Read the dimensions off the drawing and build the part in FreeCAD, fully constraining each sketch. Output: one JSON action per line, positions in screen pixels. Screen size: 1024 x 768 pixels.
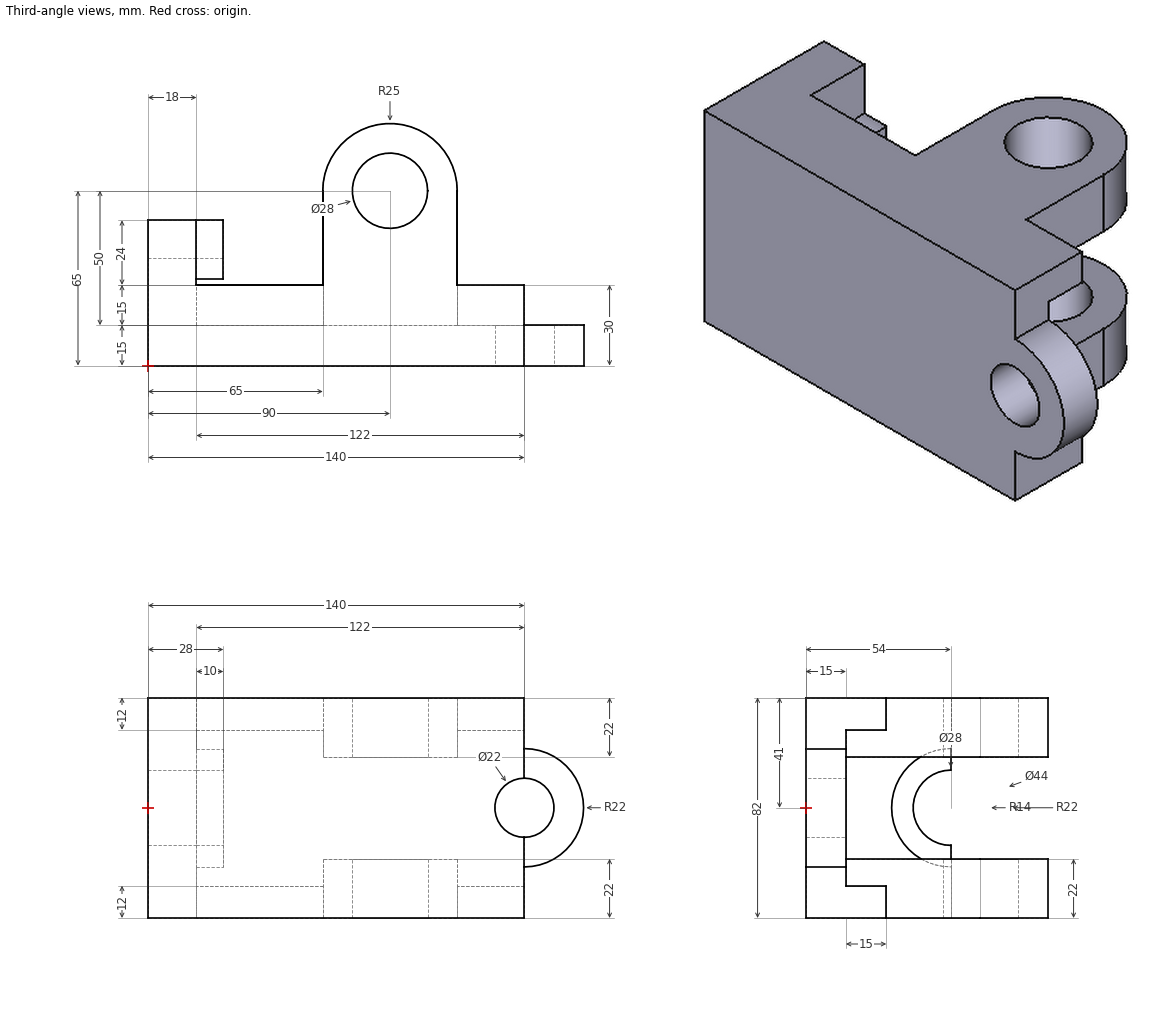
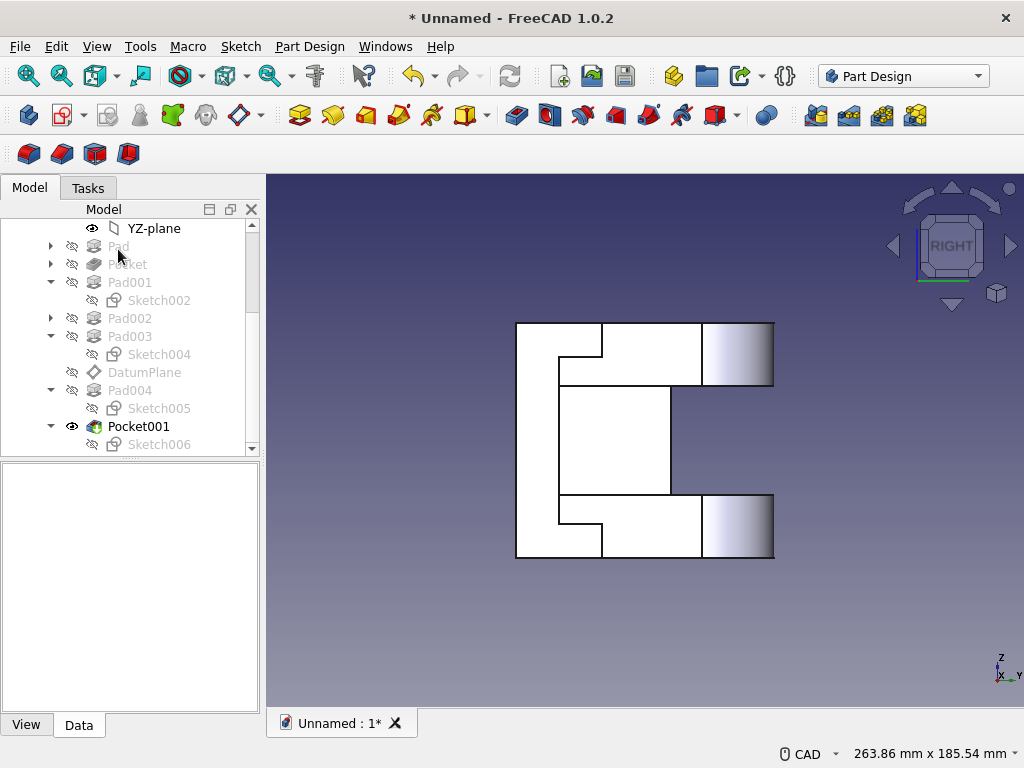
{"action": "left_click", "coordinate": [615, 439]}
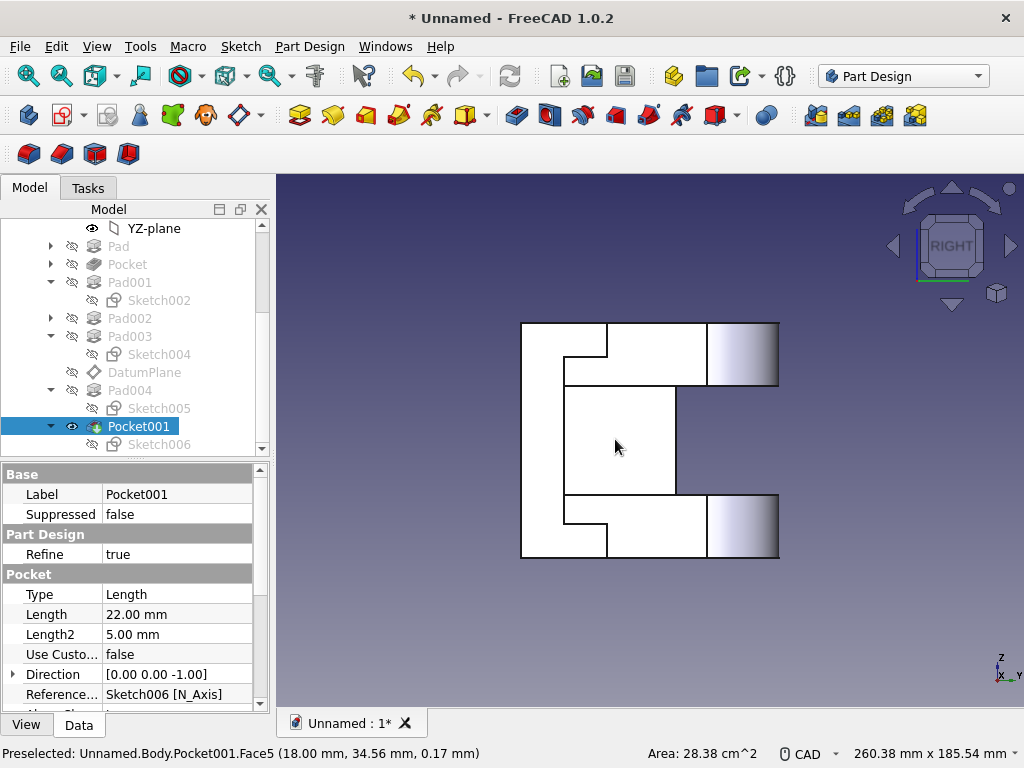
{"action": "left_click", "coordinate": [62, 116]}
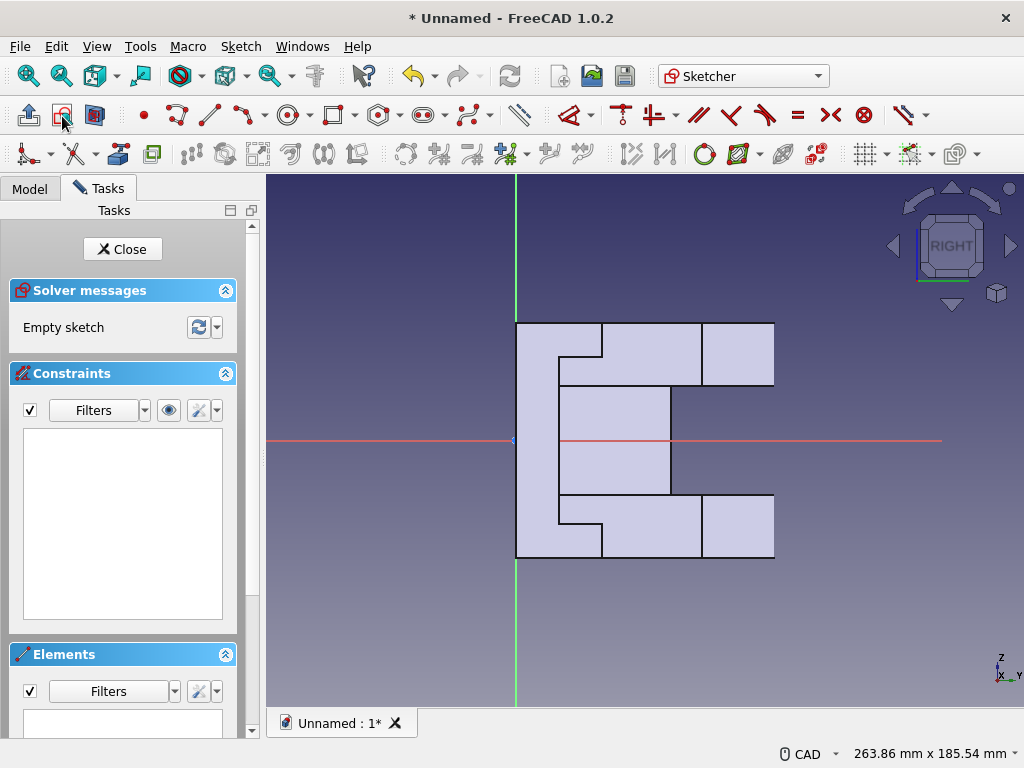
{"action": "scroll", "coordinate": [684, 441], "scroll_direction": "up", "scroll_amount": 3}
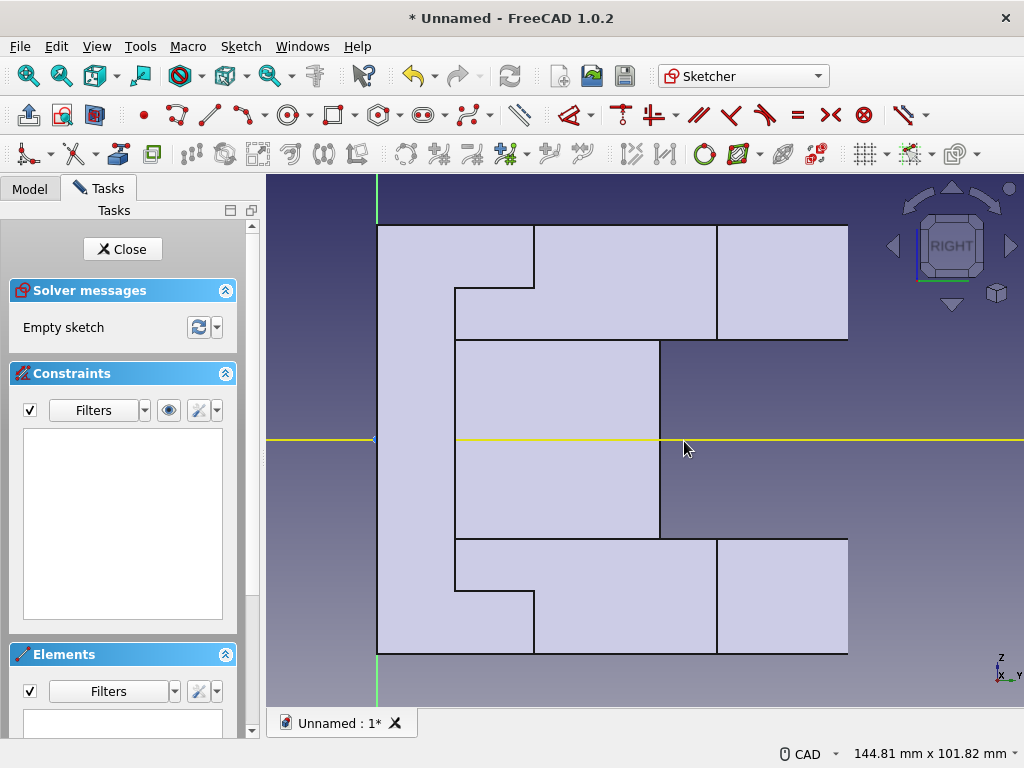
{"action": "left_click", "coordinate": [288, 116]}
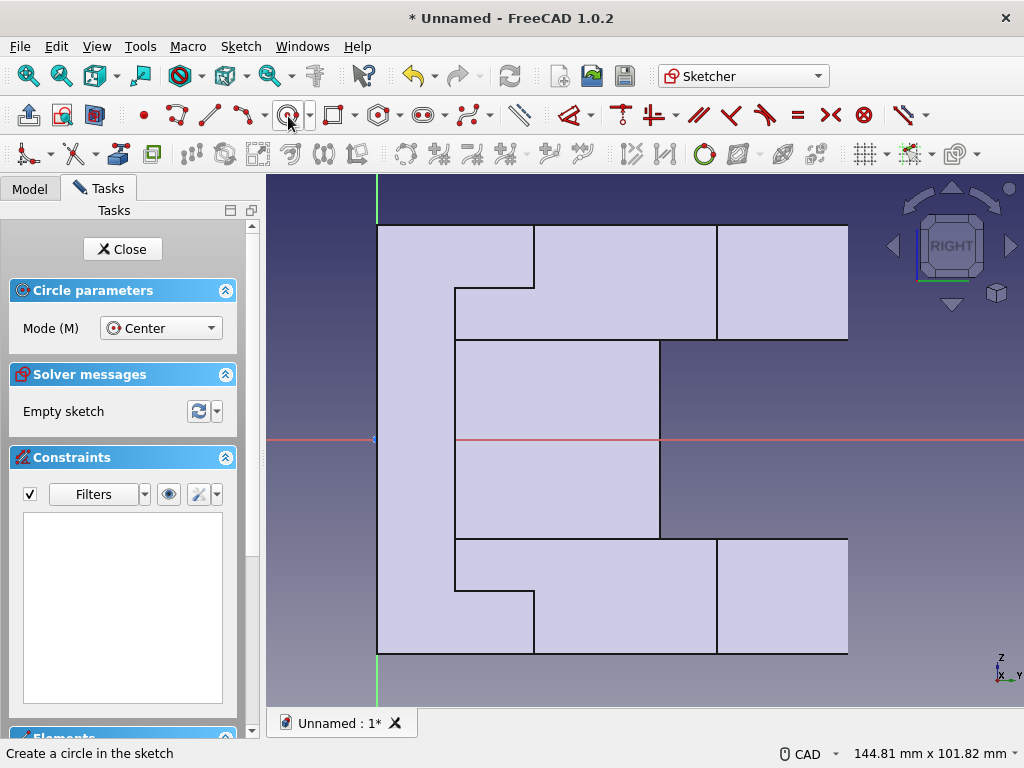
{"action": "left_click", "coordinate": [660, 440]}
{"action": "left_click", "coordinate": [741, 358]}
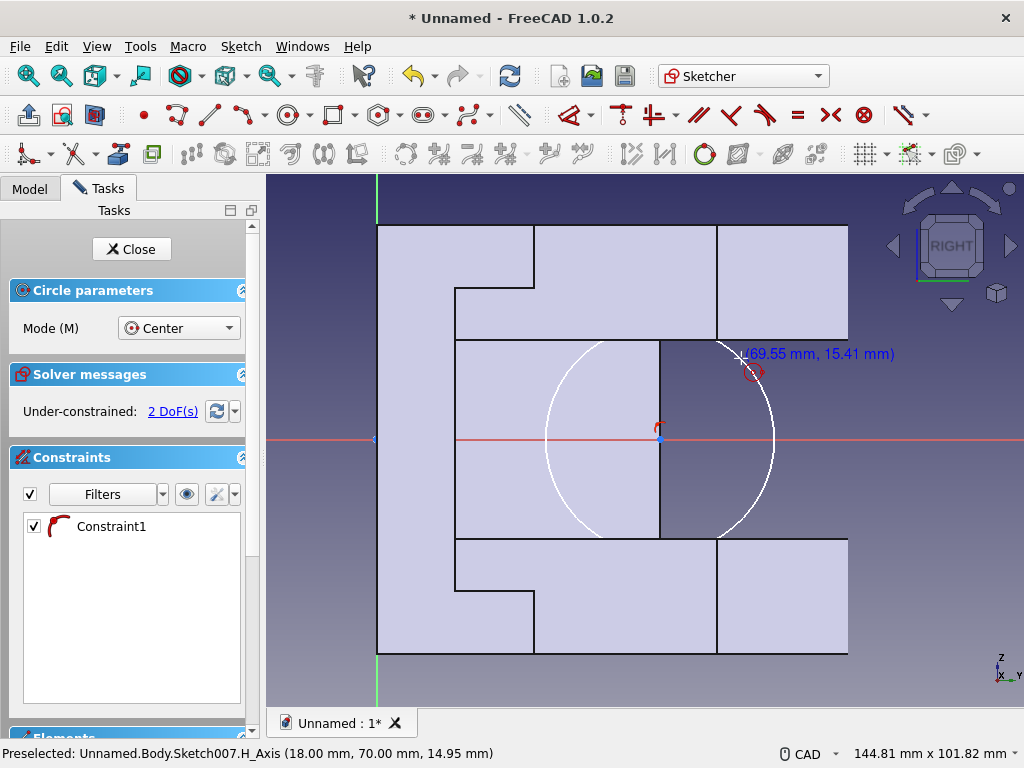
{"action": "left_click", "coordinate": [660, 440]}
{"action": "left_click", "coordinate": [711, 388]}
{"action": "key", "text": "Escape"}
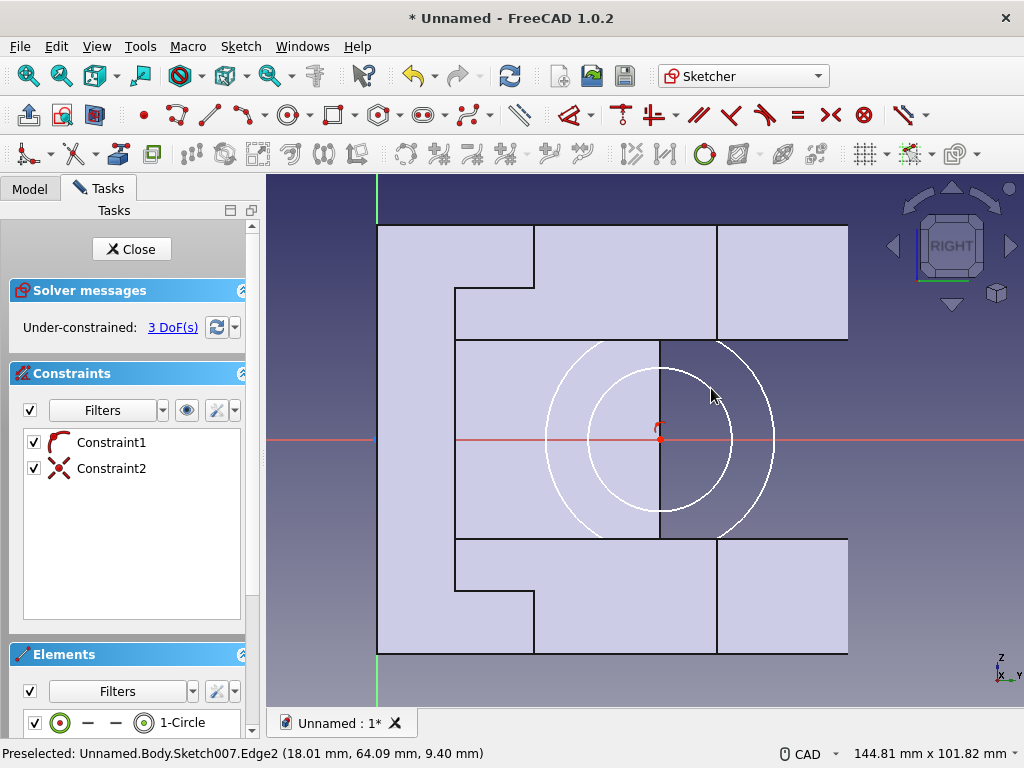
{"action": "key", "text": "d"}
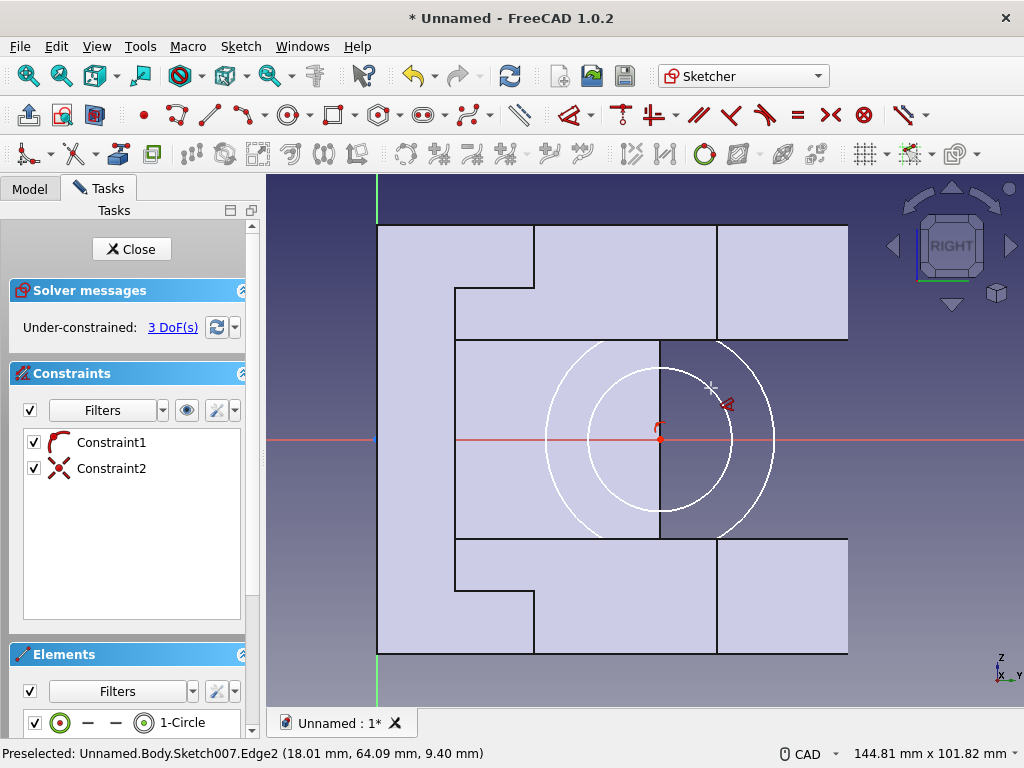
{"action": "left_click", "coordinate": [741, 359]}
{"action": "left_click", "coordinate": [764, 336]}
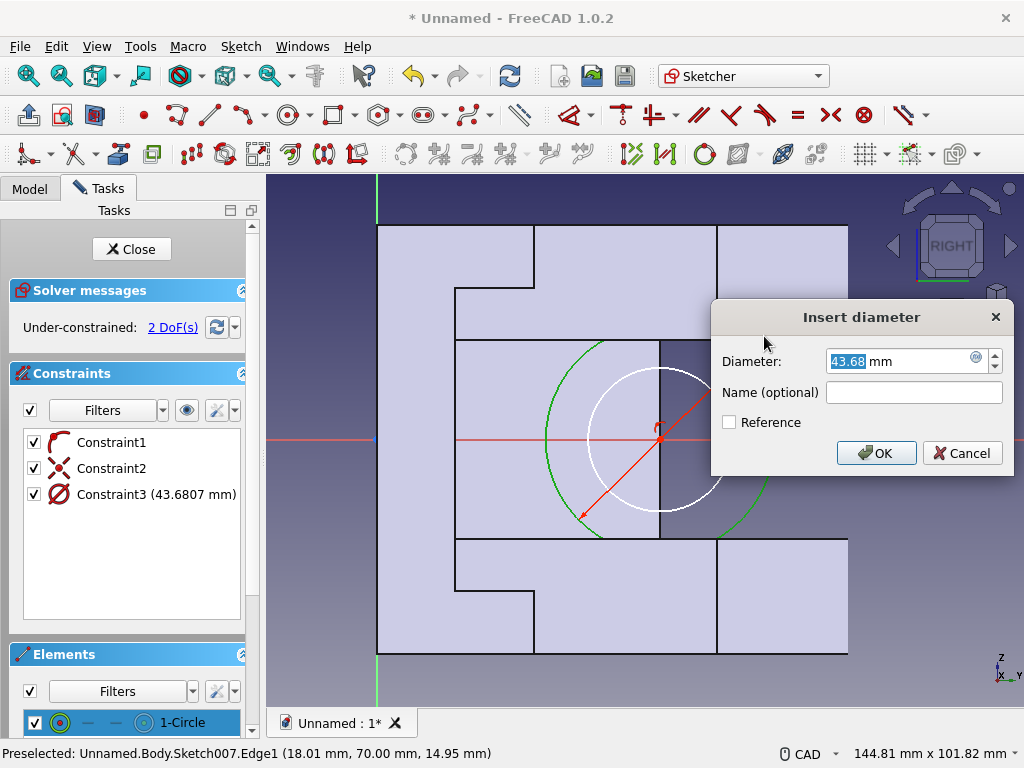
{"action": "type", "text": "44"}
{"action": "key", "text": "Return"}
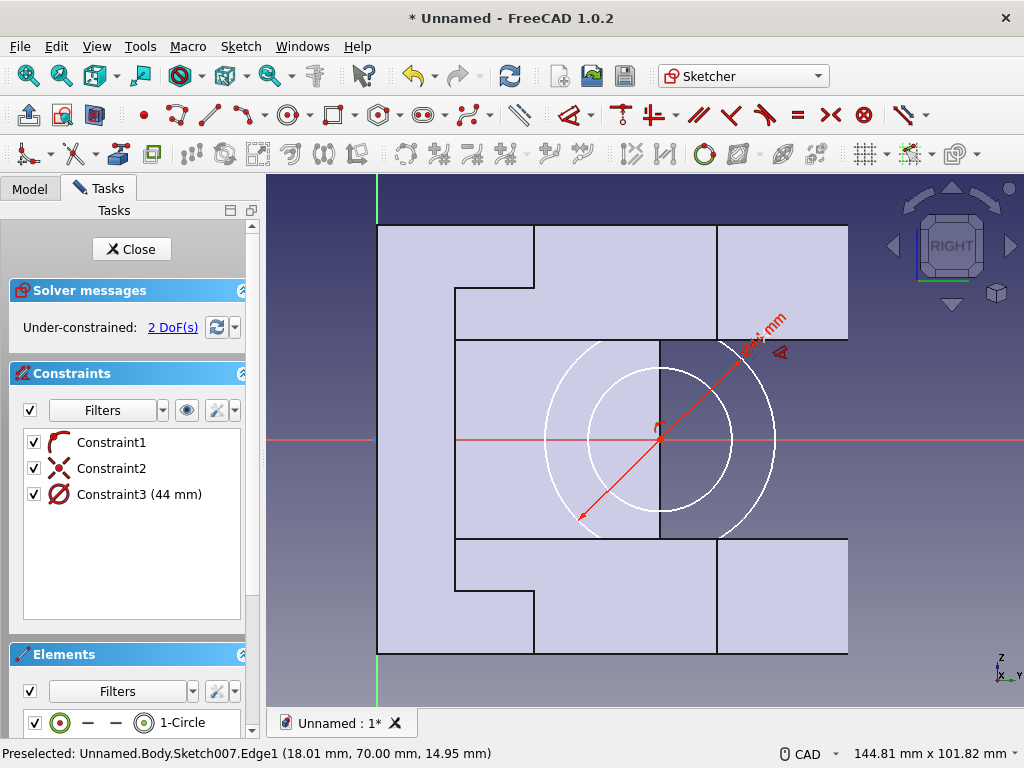
{"action": "left_click", "coordinate": [711, 389]}
{"action": "left_click", "coordinate": [806, 397]}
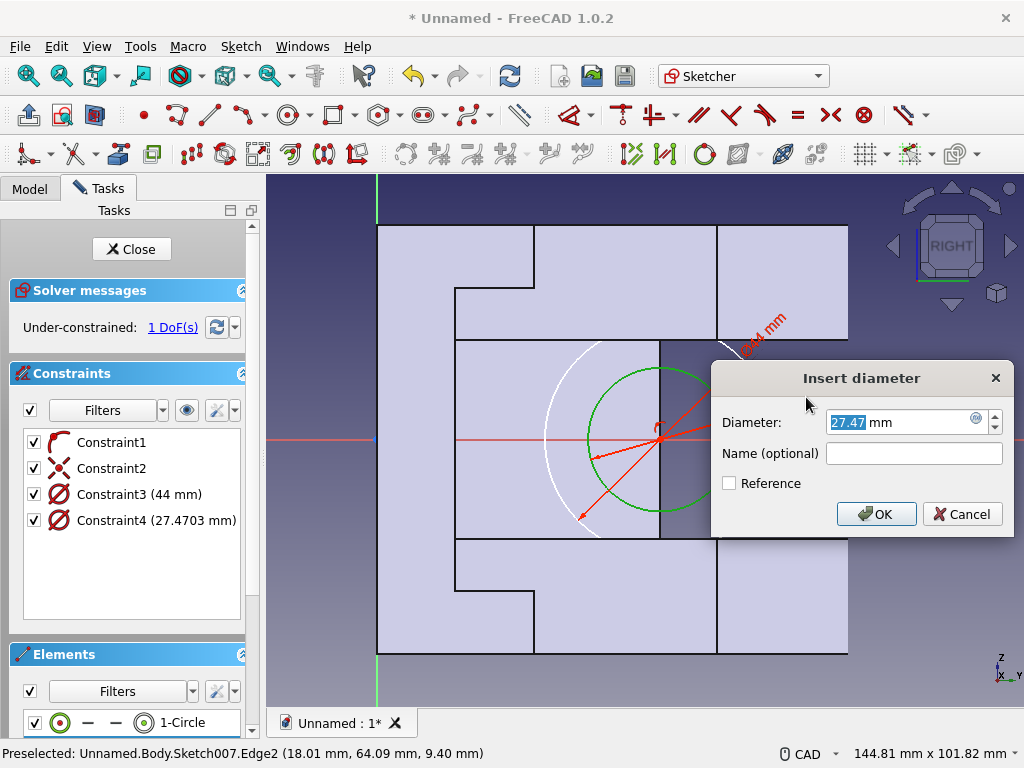
{"action": "type", "text": "28"}
{"action": "key", "text": "Return"}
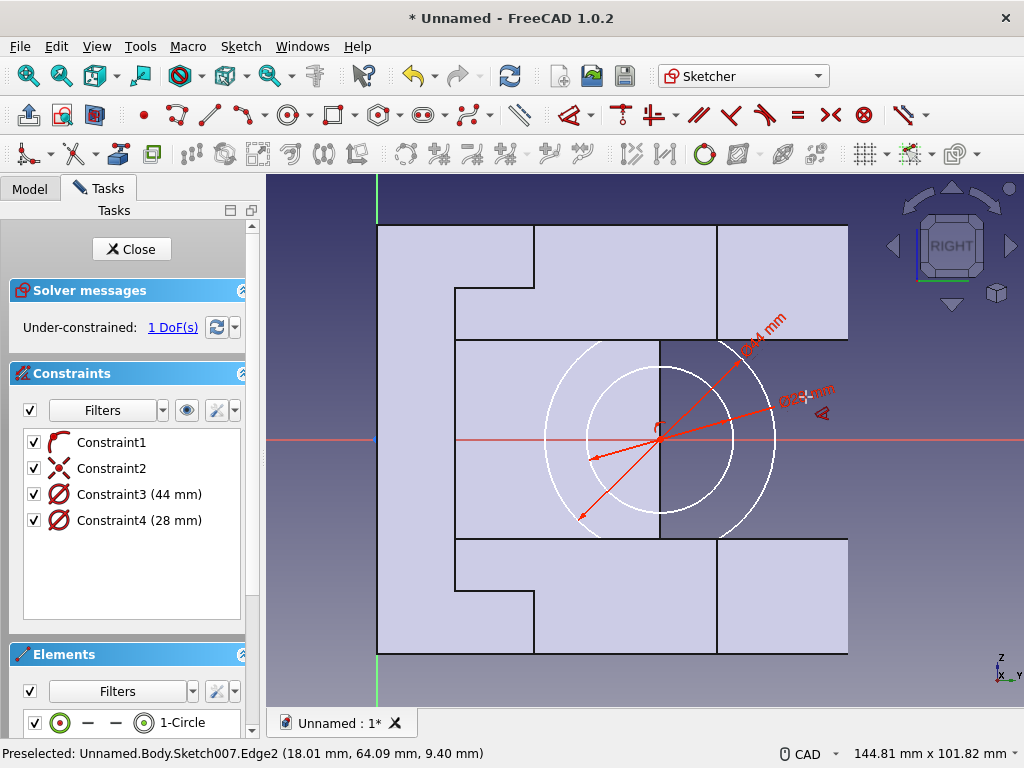
{"action": "left_click", "coordinate": [660, 440]}
{"action": "left_click", "coordinate": [518, 474]}